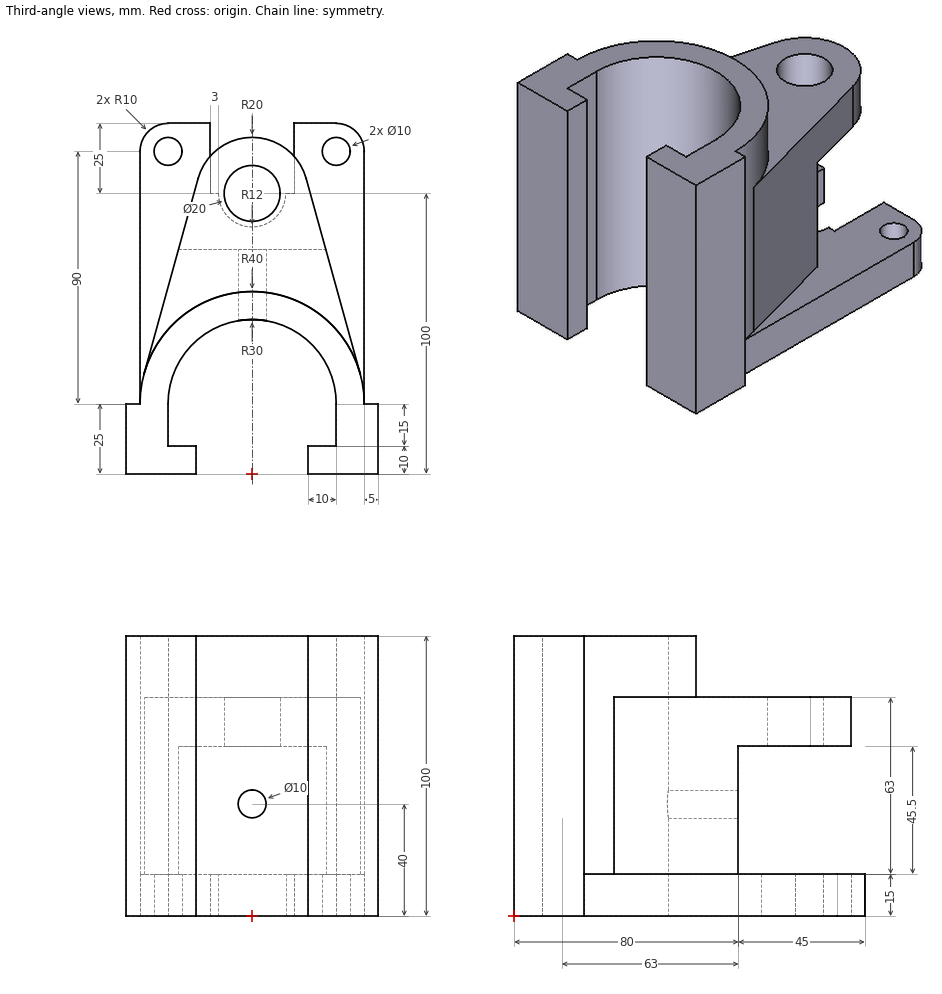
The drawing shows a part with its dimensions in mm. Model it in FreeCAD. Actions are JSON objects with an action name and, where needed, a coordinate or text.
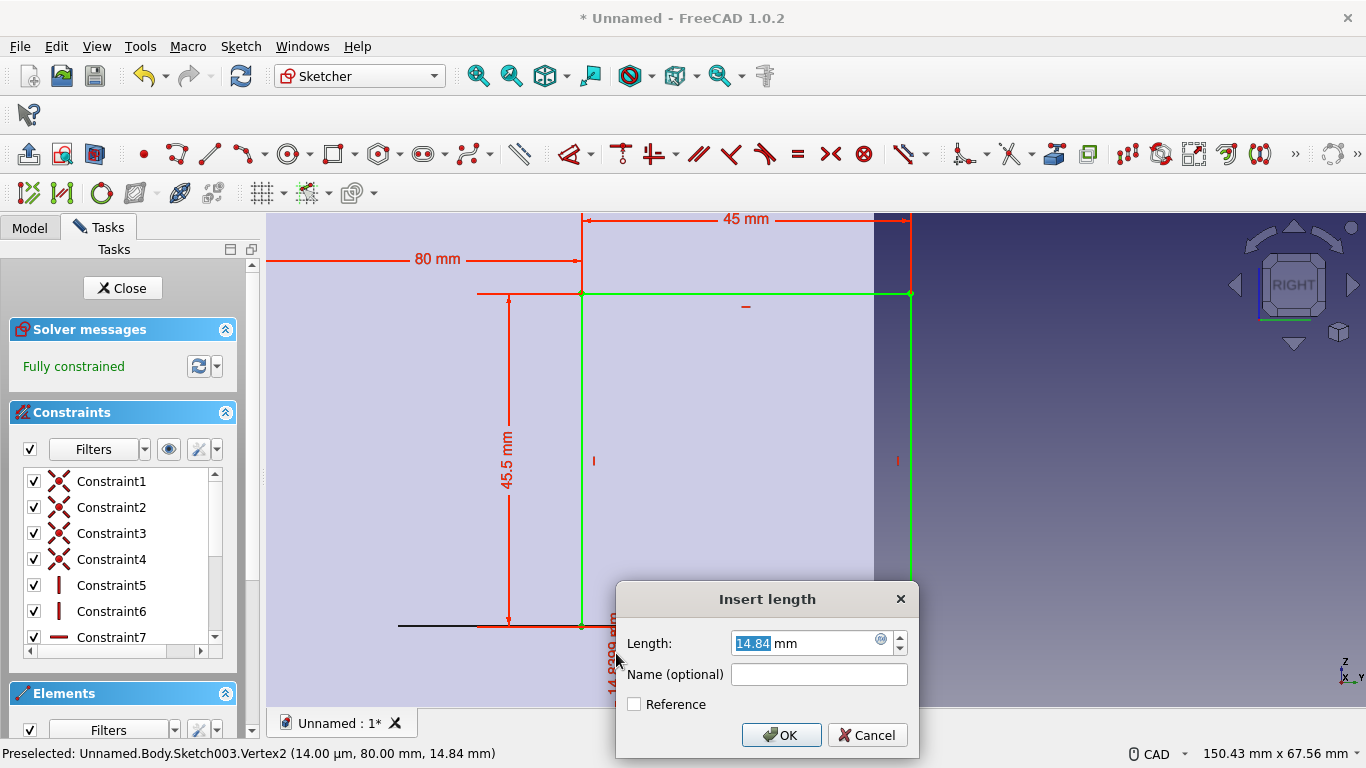
{"action": "type", "text": "15"}
{"action": "key", "text": "Return"}
{"action": "key", "text": "Escape"}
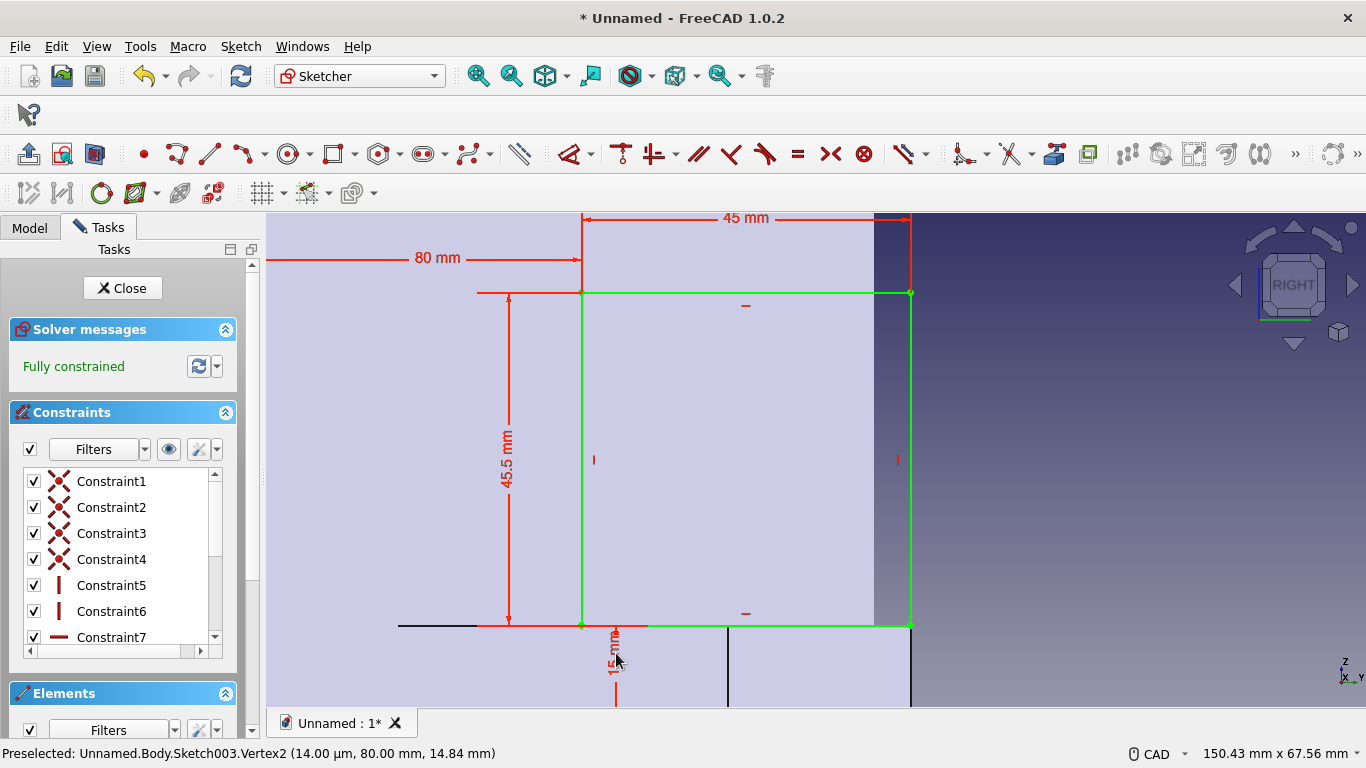
{"action": "left_click", "coordinate": [123, 288]}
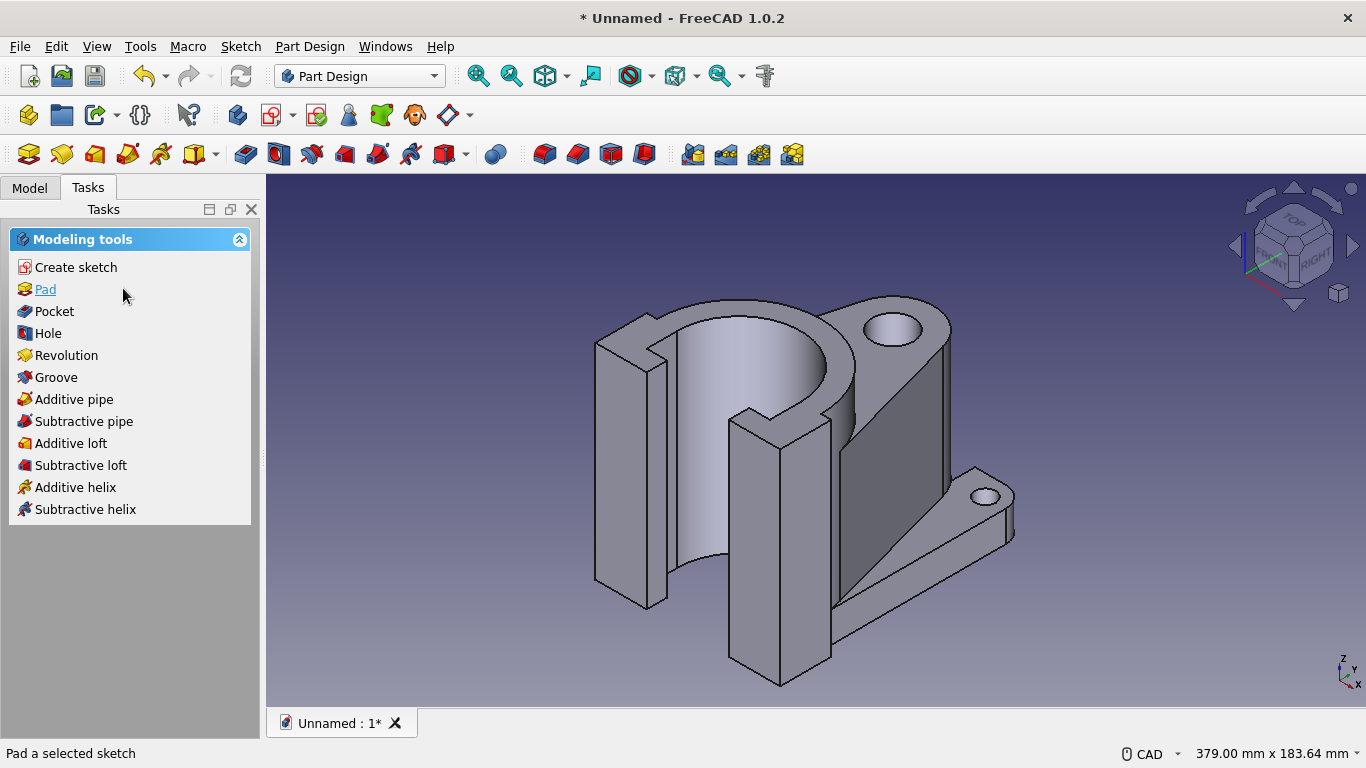
{"action": "left_click", "coordinate": [246, 154]}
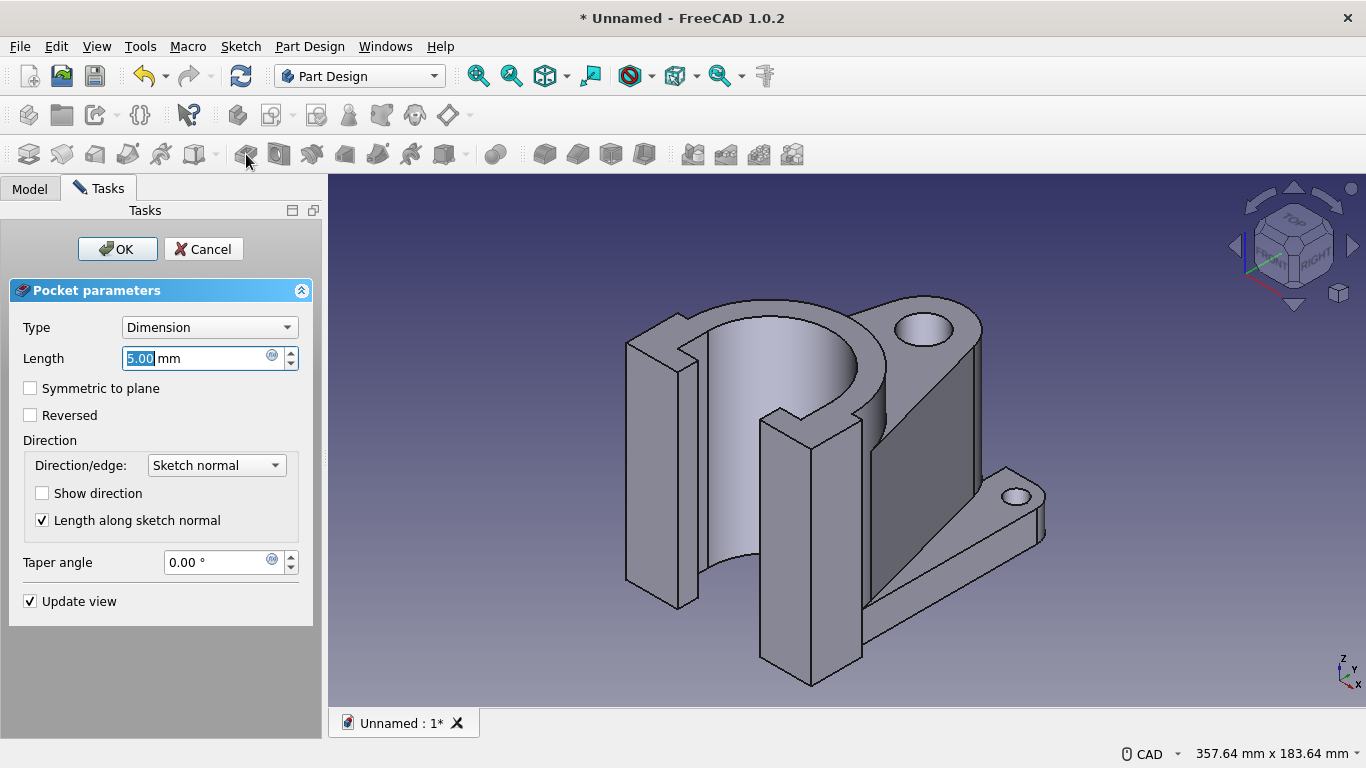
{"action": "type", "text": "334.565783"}
{"action": "key", "text": "Tab"}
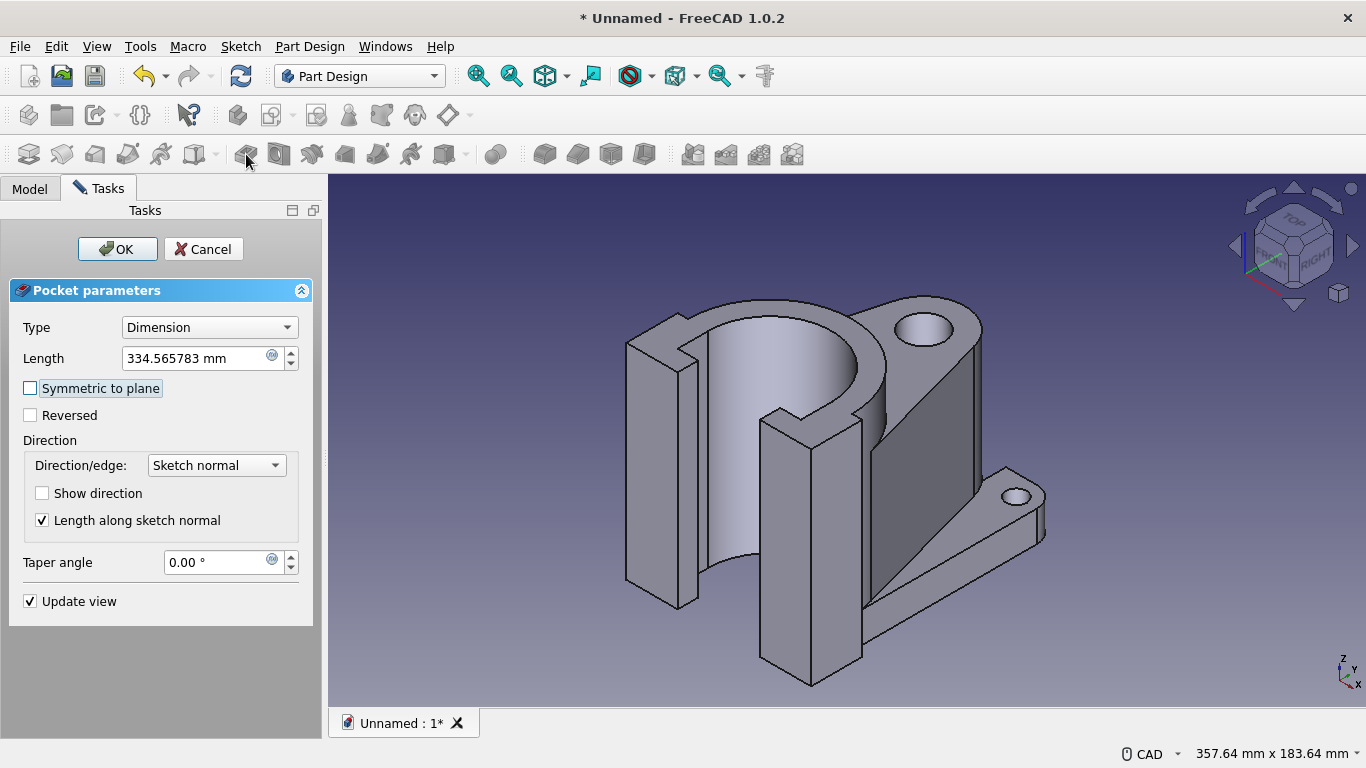
{"action": "left_click", "coordinate": [31, 388]}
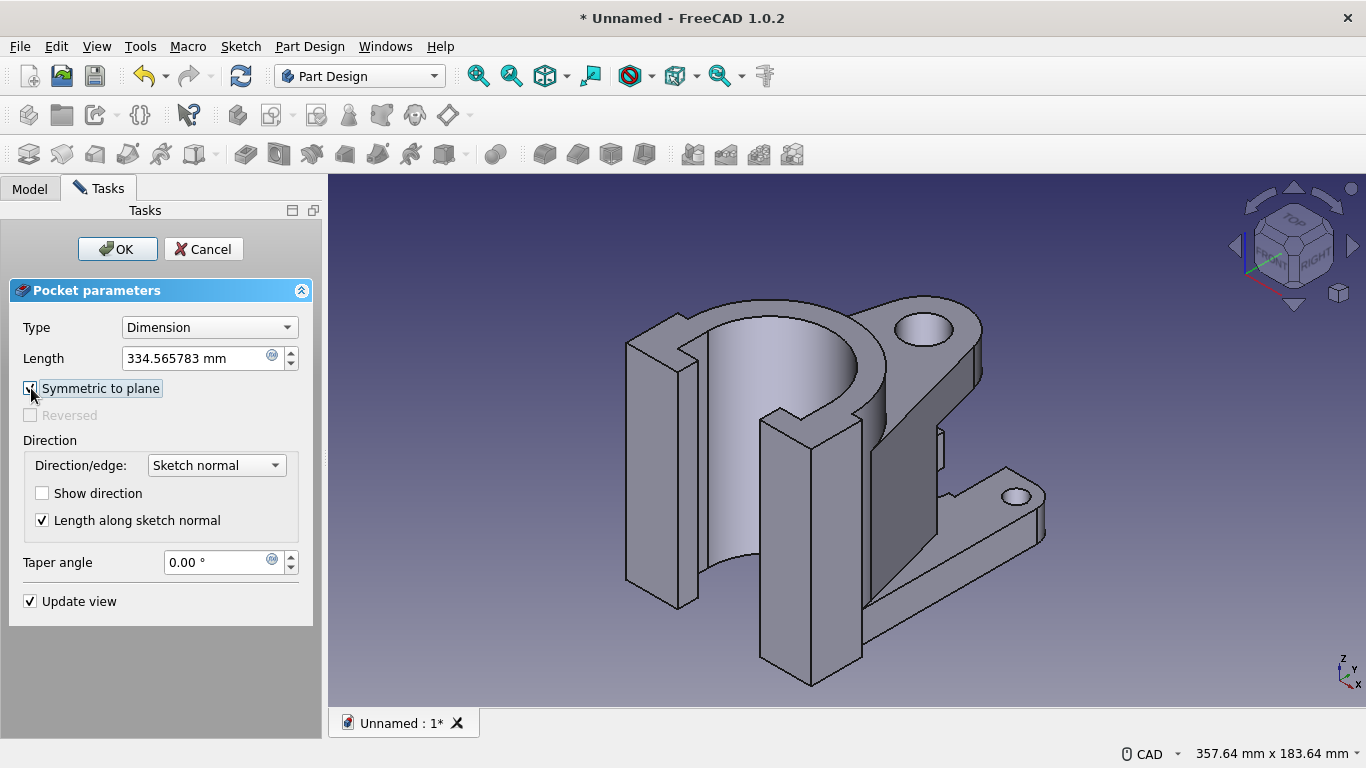
{"action": "left_click", "coordinate": [118, 249]}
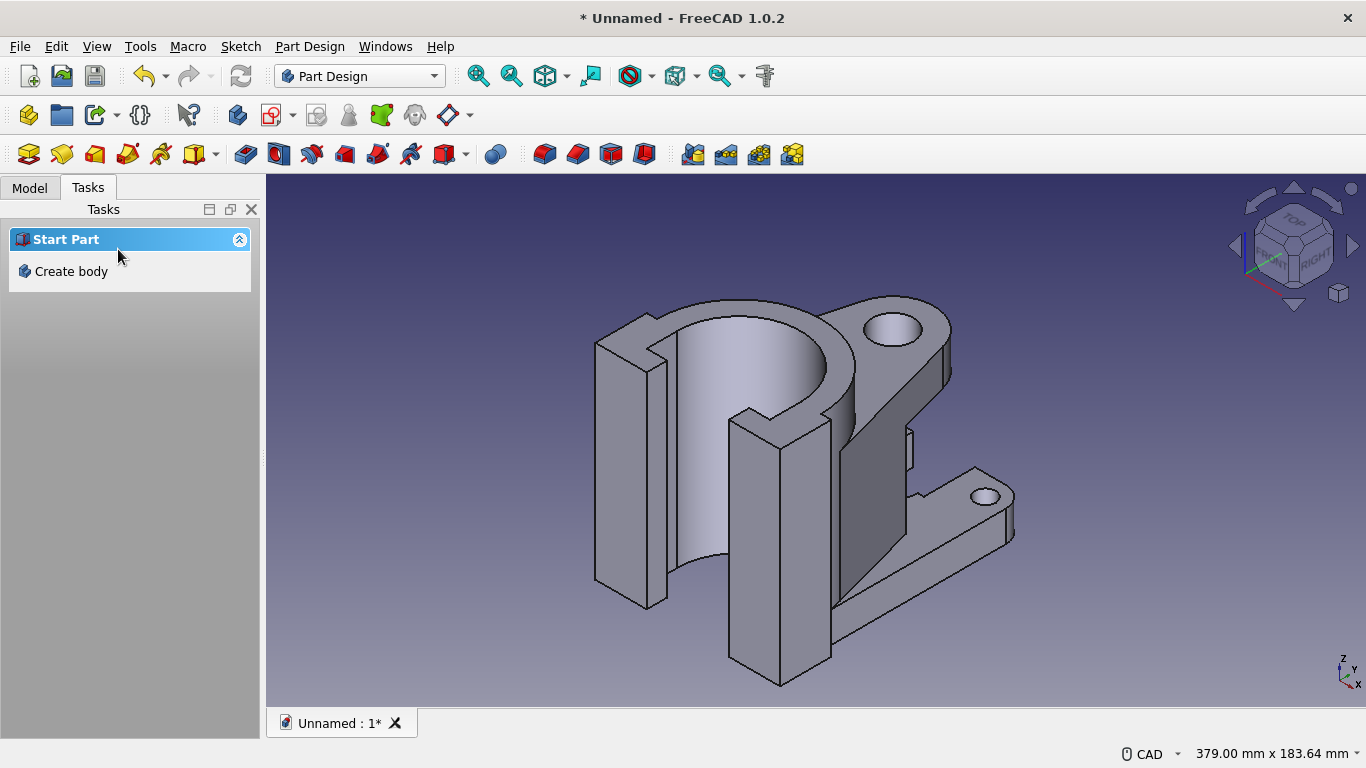
{"action": "key", "text": "4"}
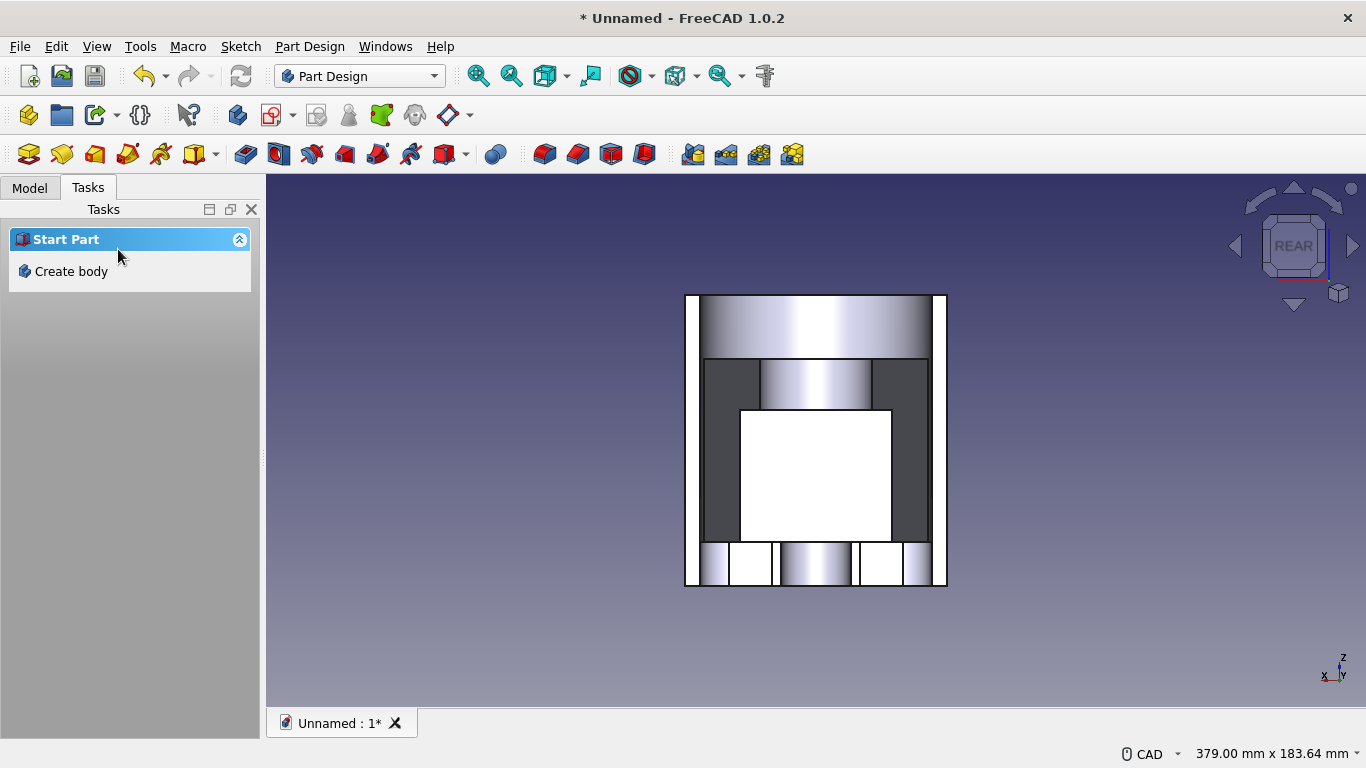
{"action": "left_click", "coordinate": [816, 475]}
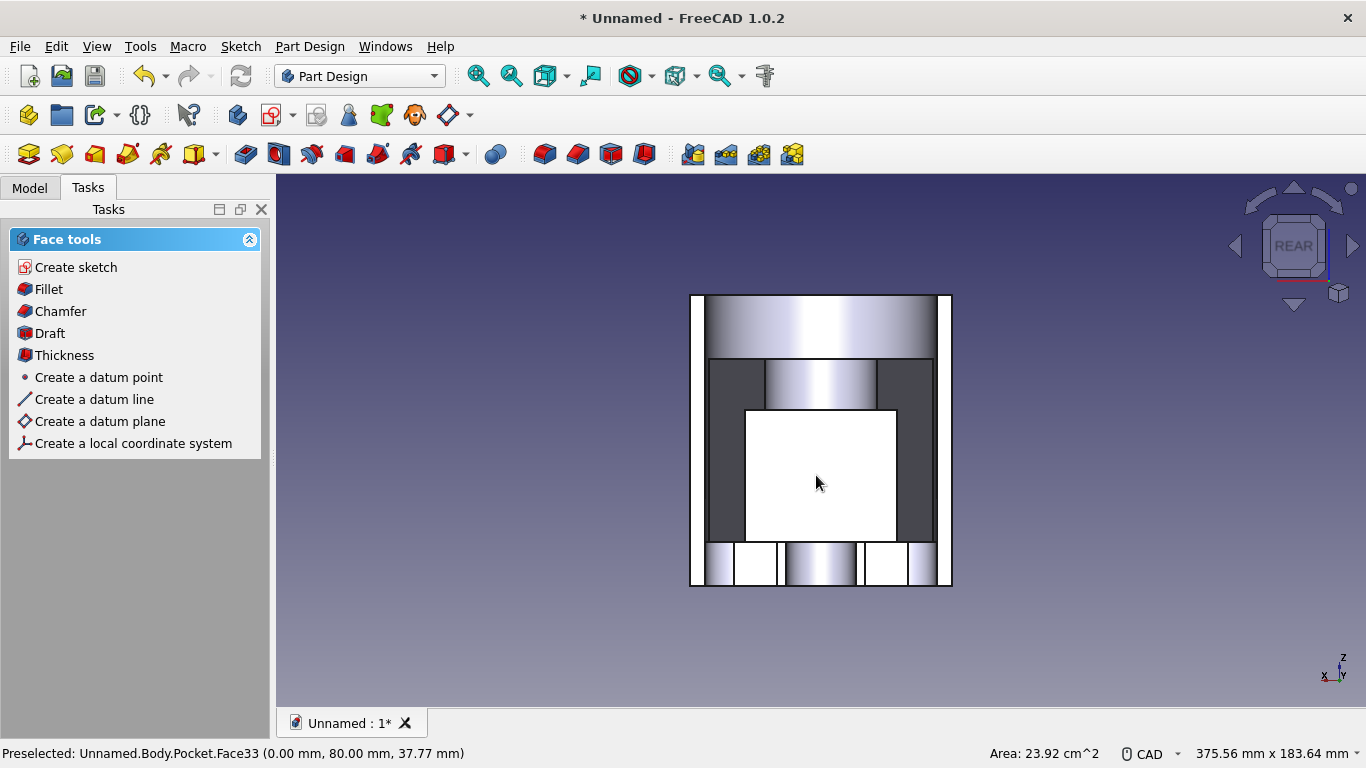
{"action": "left_click", "coordinate": [270, 116]}